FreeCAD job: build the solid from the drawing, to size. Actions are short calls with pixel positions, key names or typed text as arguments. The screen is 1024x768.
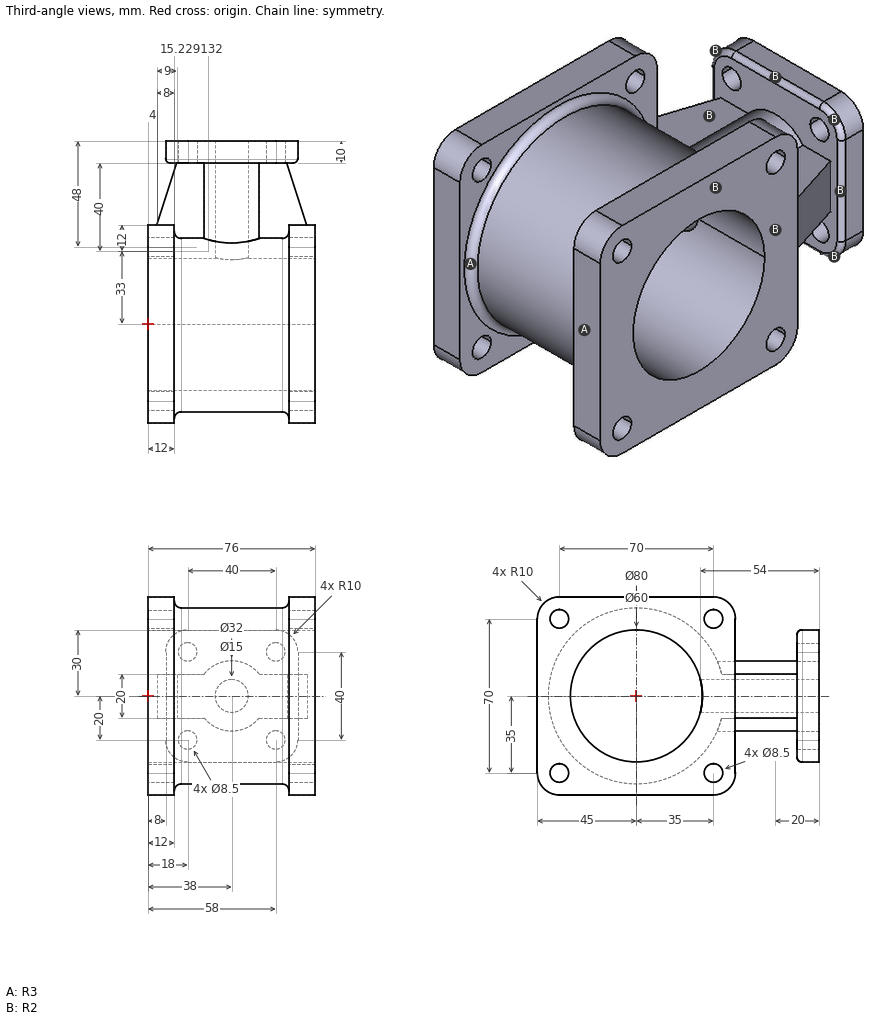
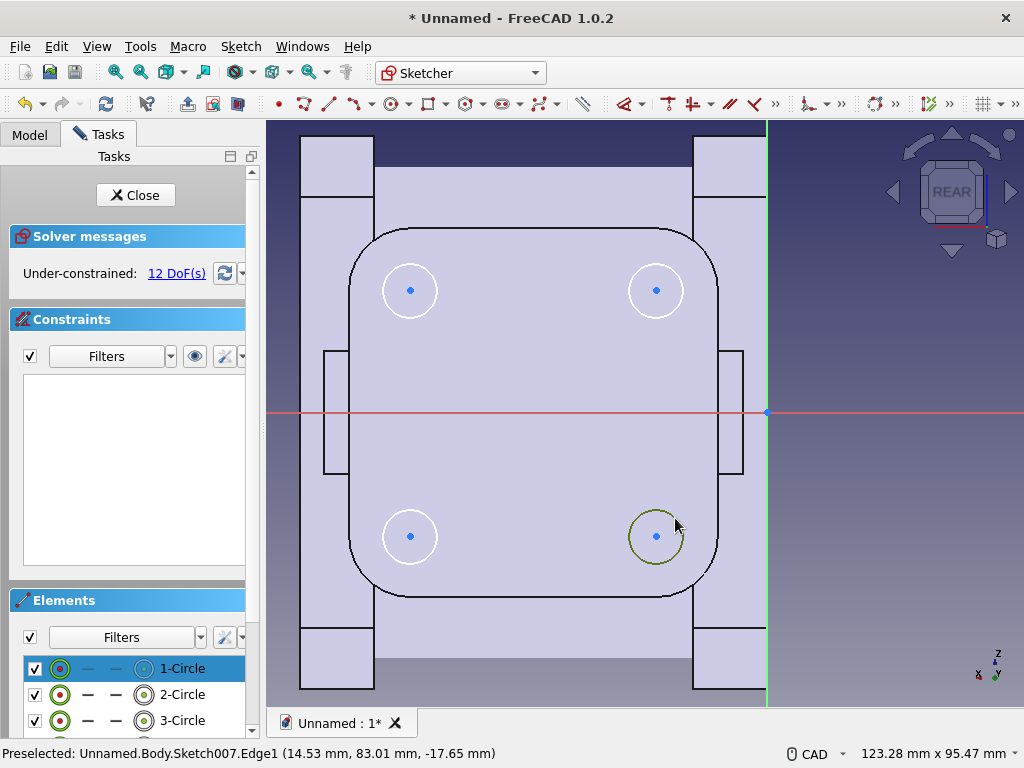
click(429, 518)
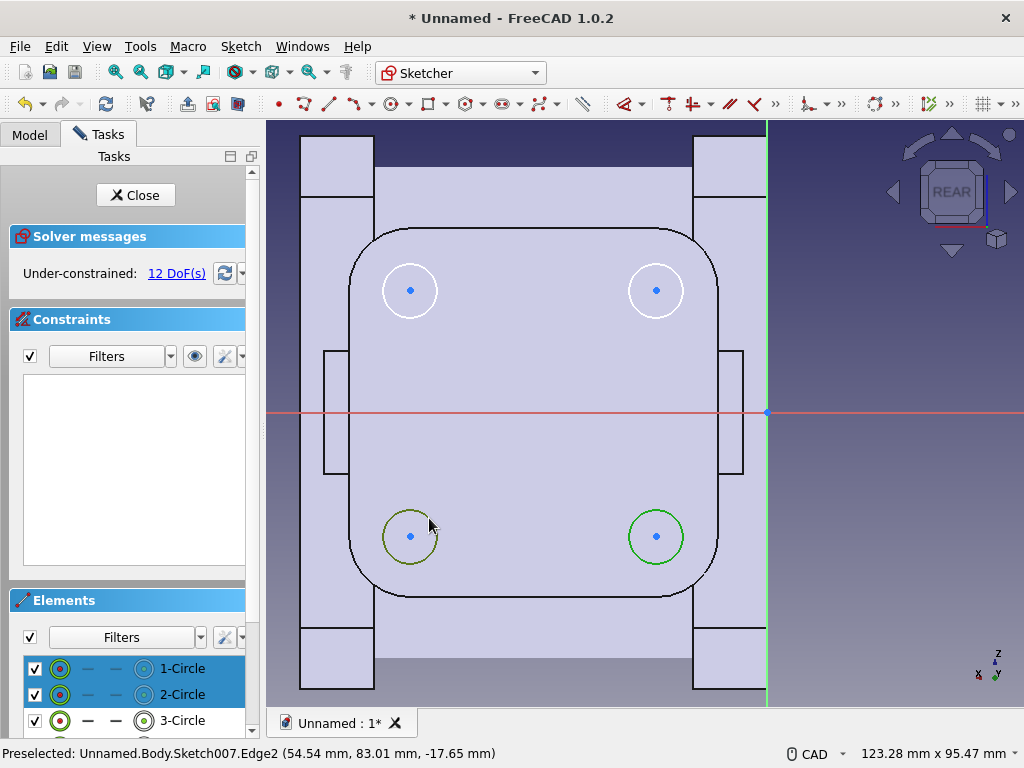
click(675, 272)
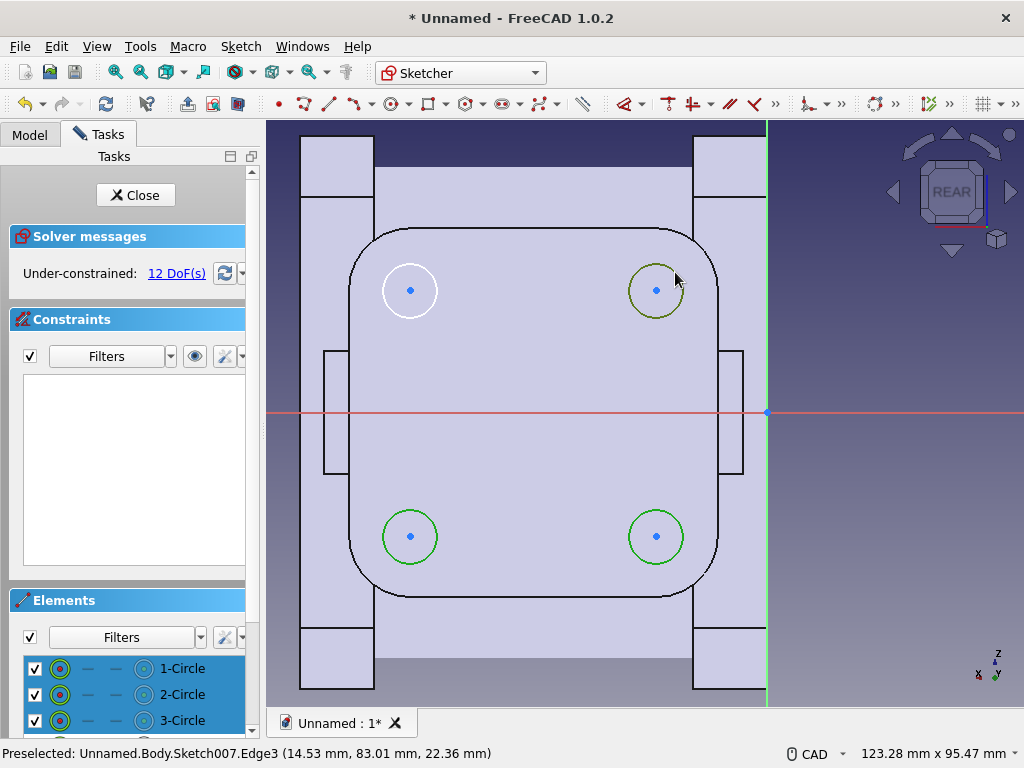
click(429, 272)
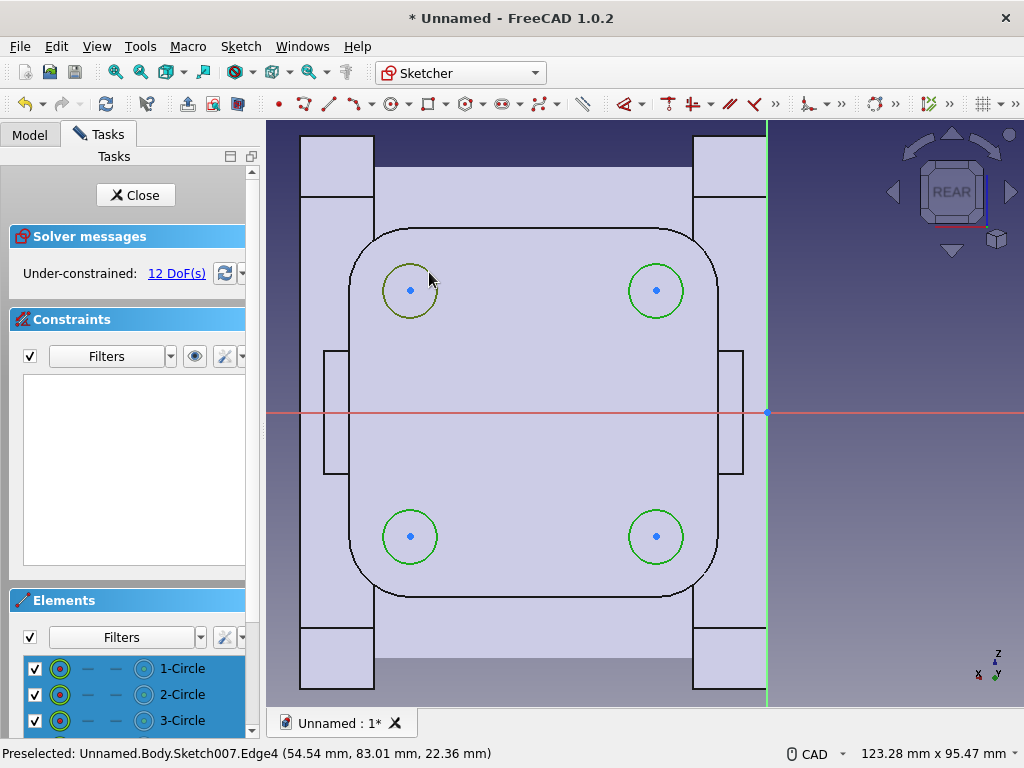
key(e)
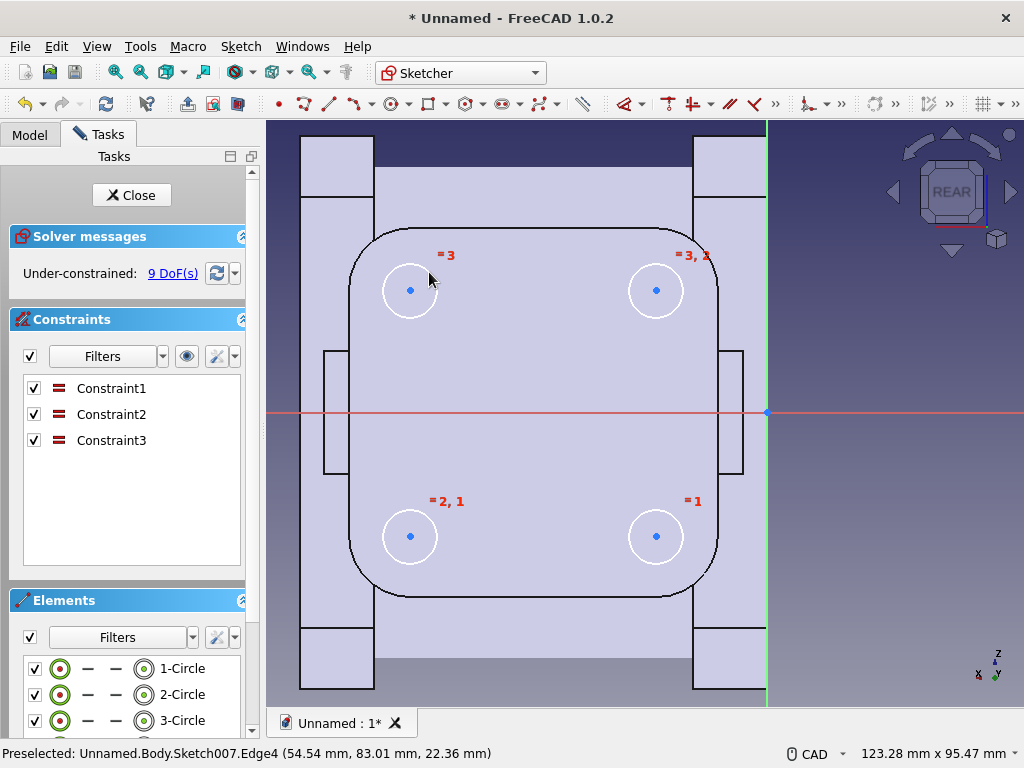
click(656, 537)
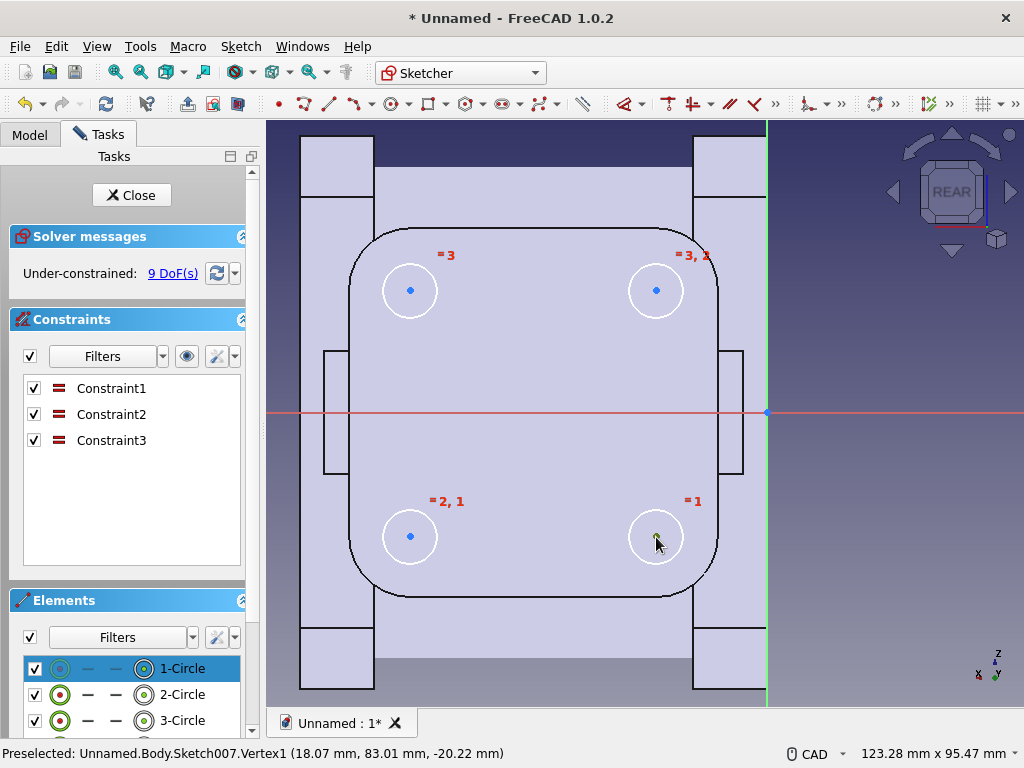
click(656, 291)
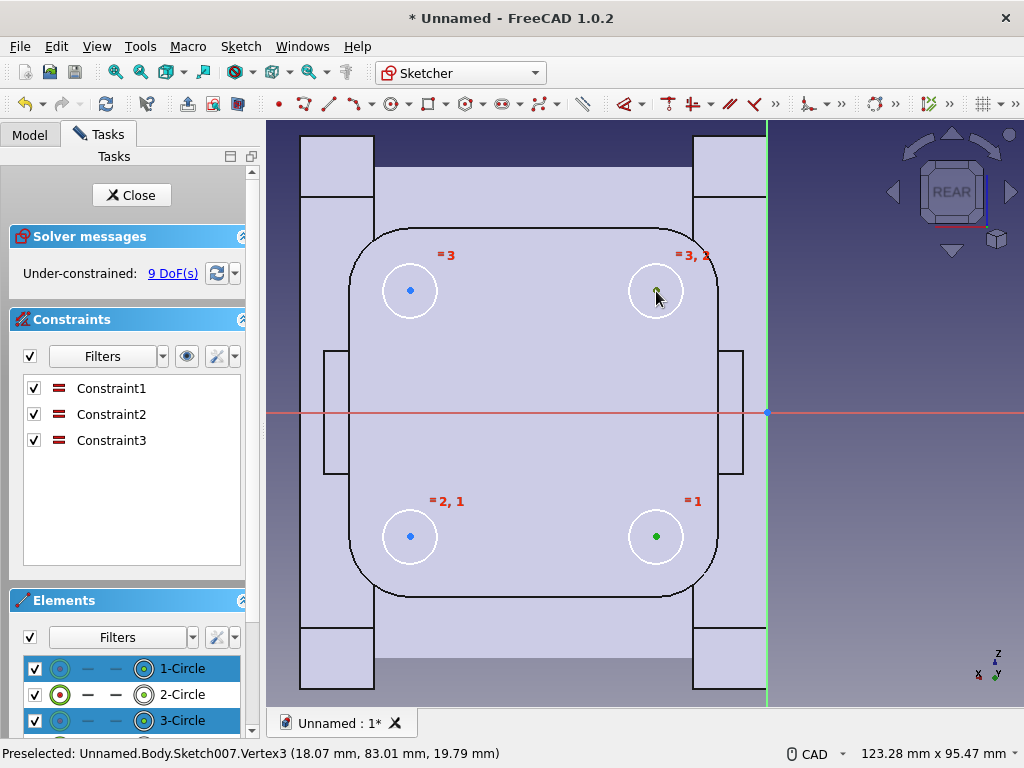
click(334, 413)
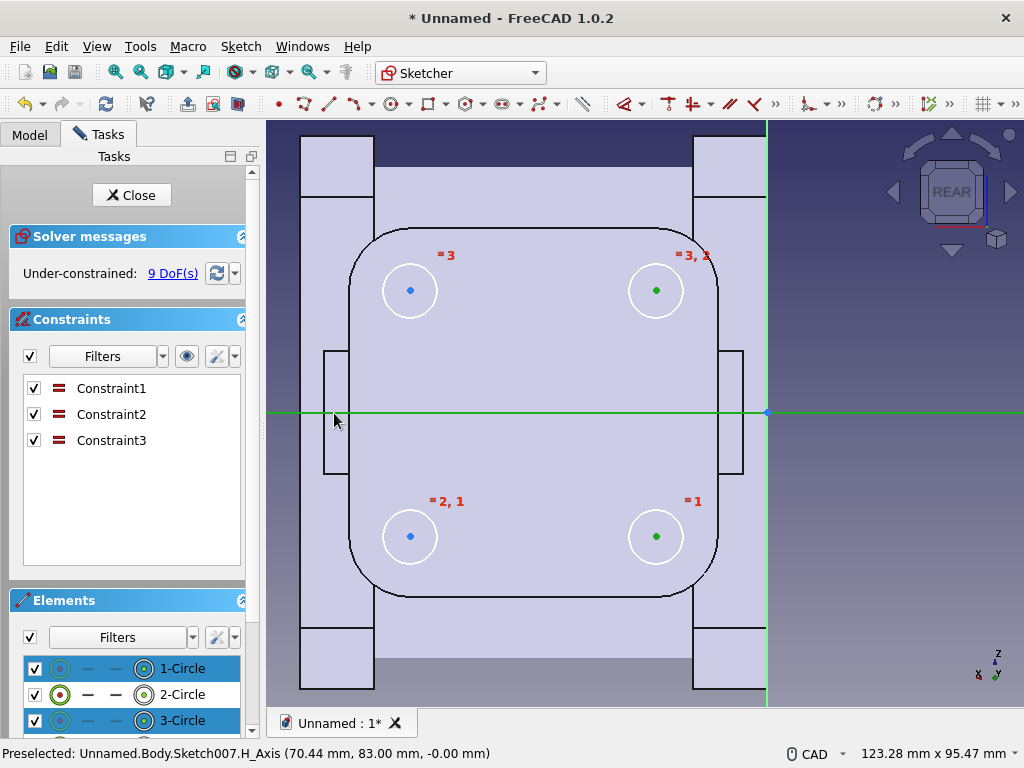
key(s)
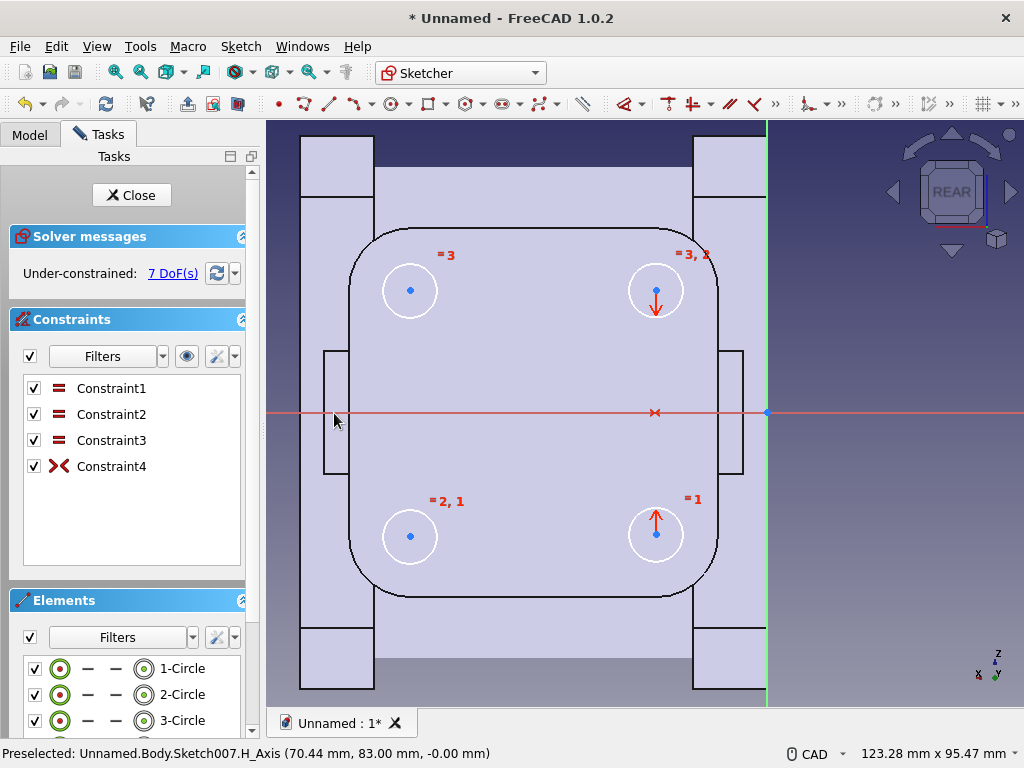
click(410, 537)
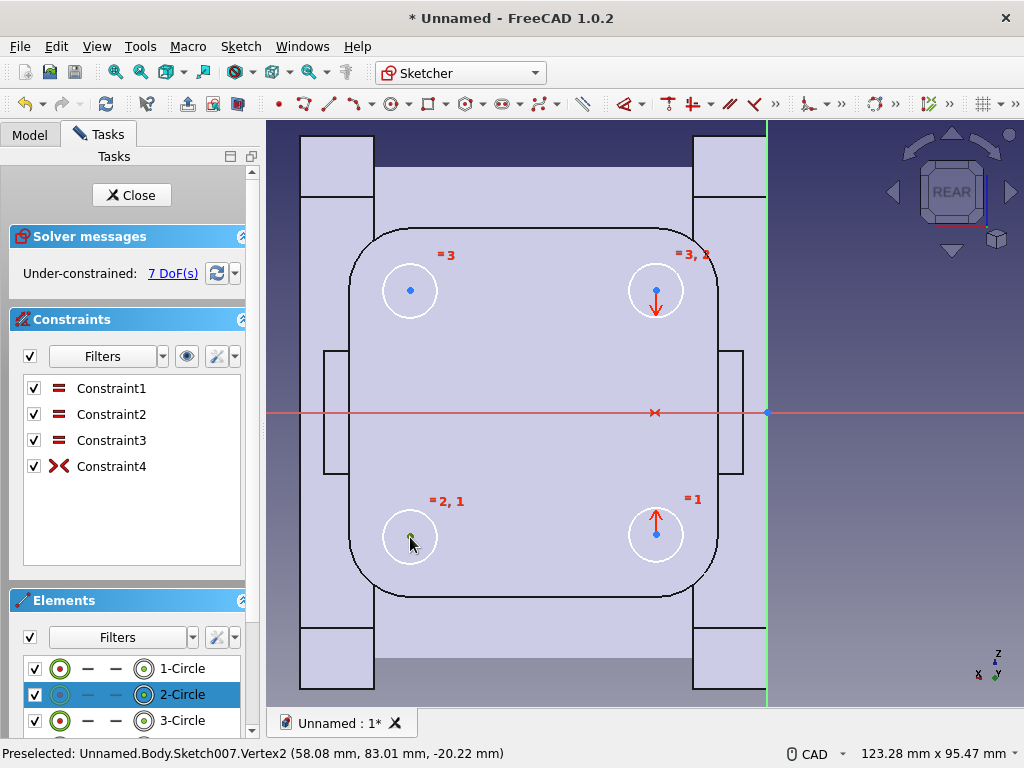
click(410, 291)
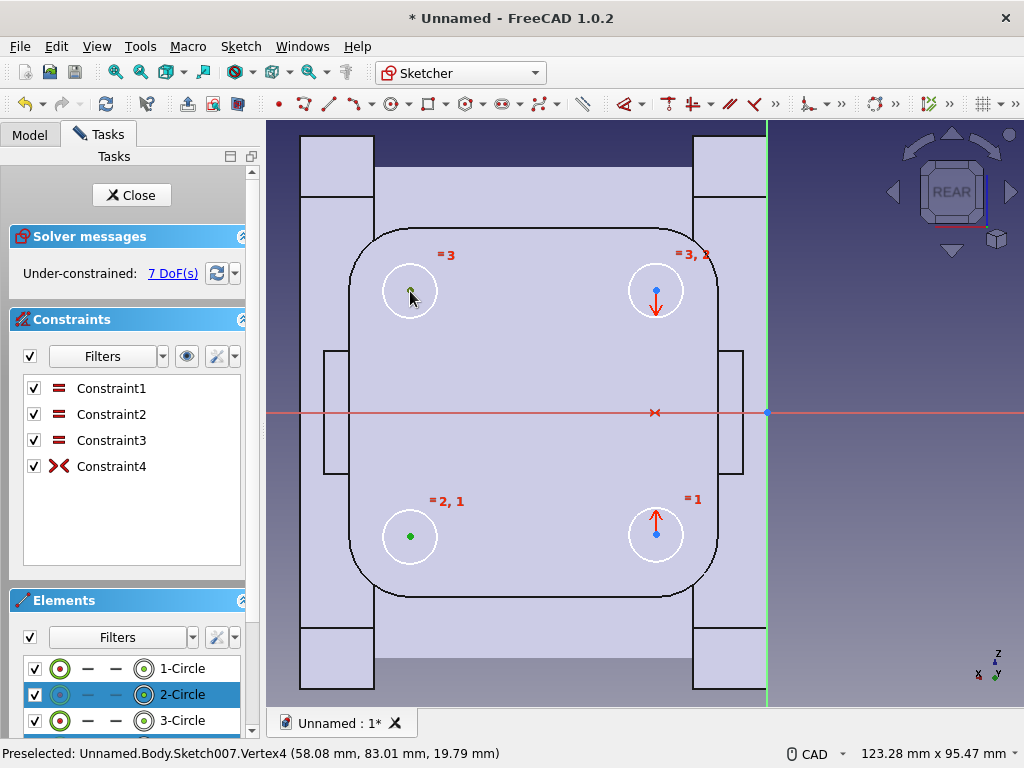
click(334, 413)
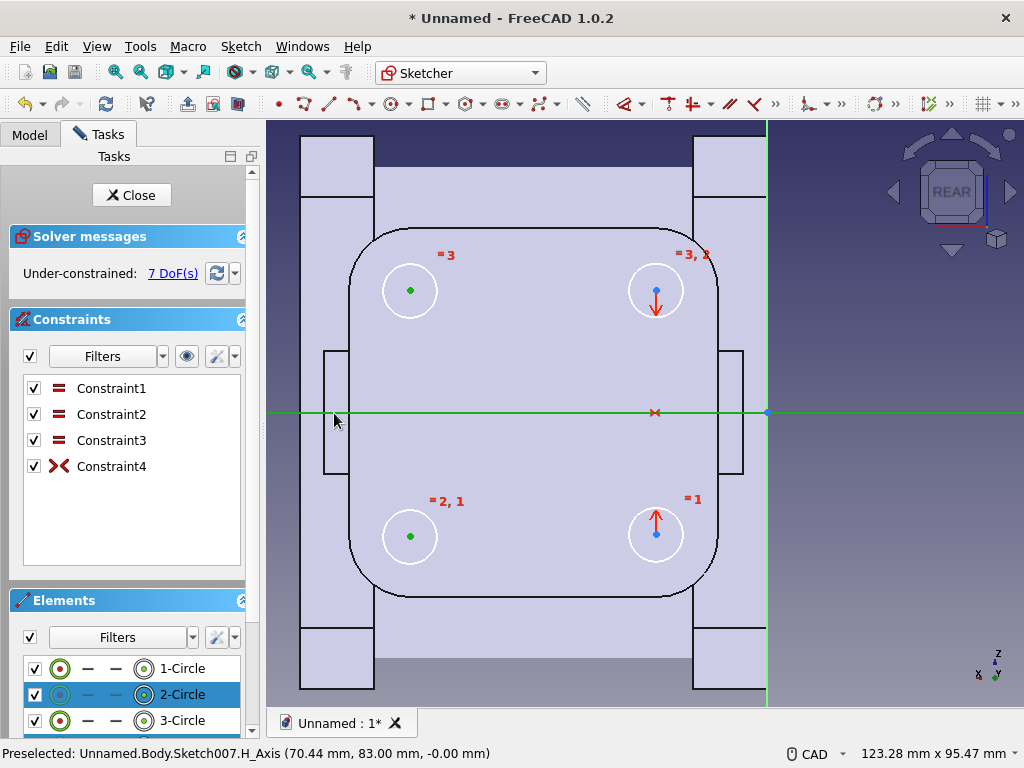
key(s)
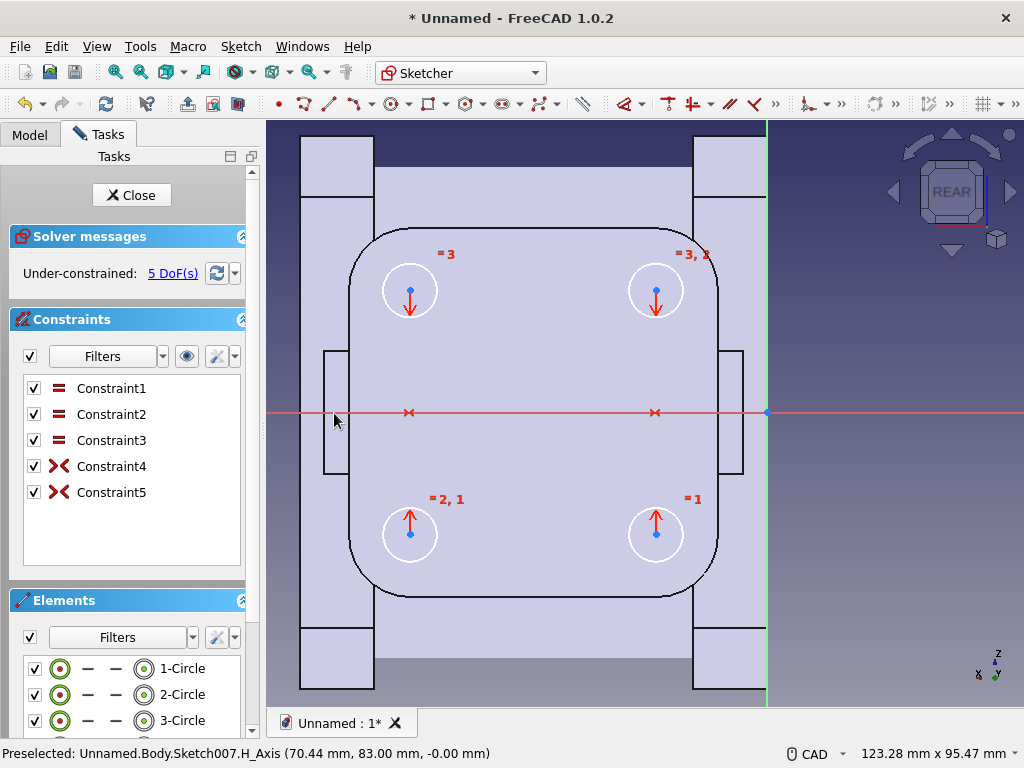
key(d)